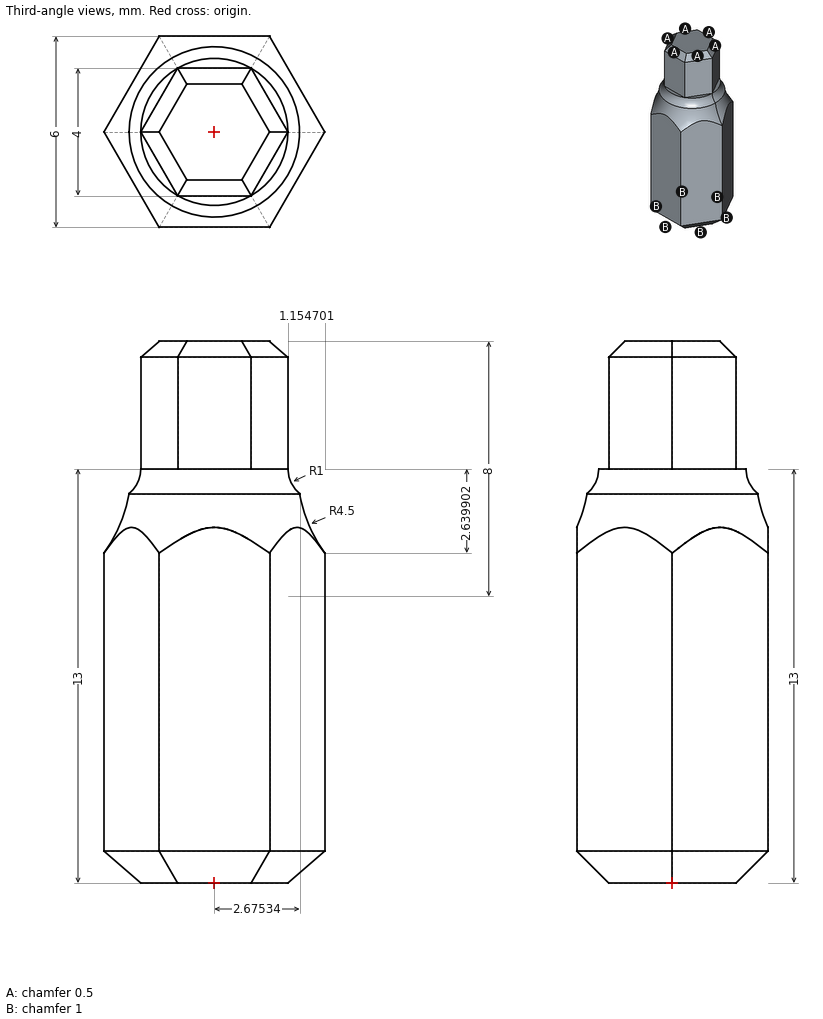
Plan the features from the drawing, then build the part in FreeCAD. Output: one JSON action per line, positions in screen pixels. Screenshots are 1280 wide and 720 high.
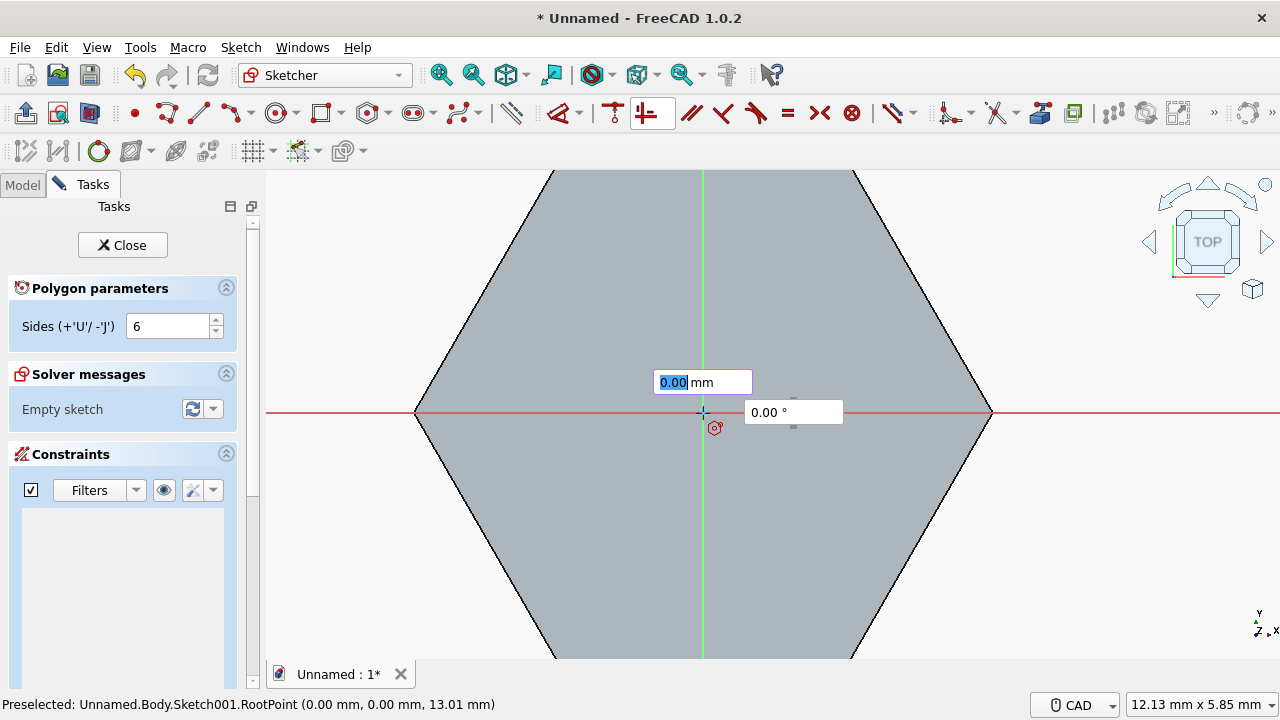
{"action": "left_click", "coordinate": [896, 413]}
{"action": "right_click", "coordinate": [896, 413]}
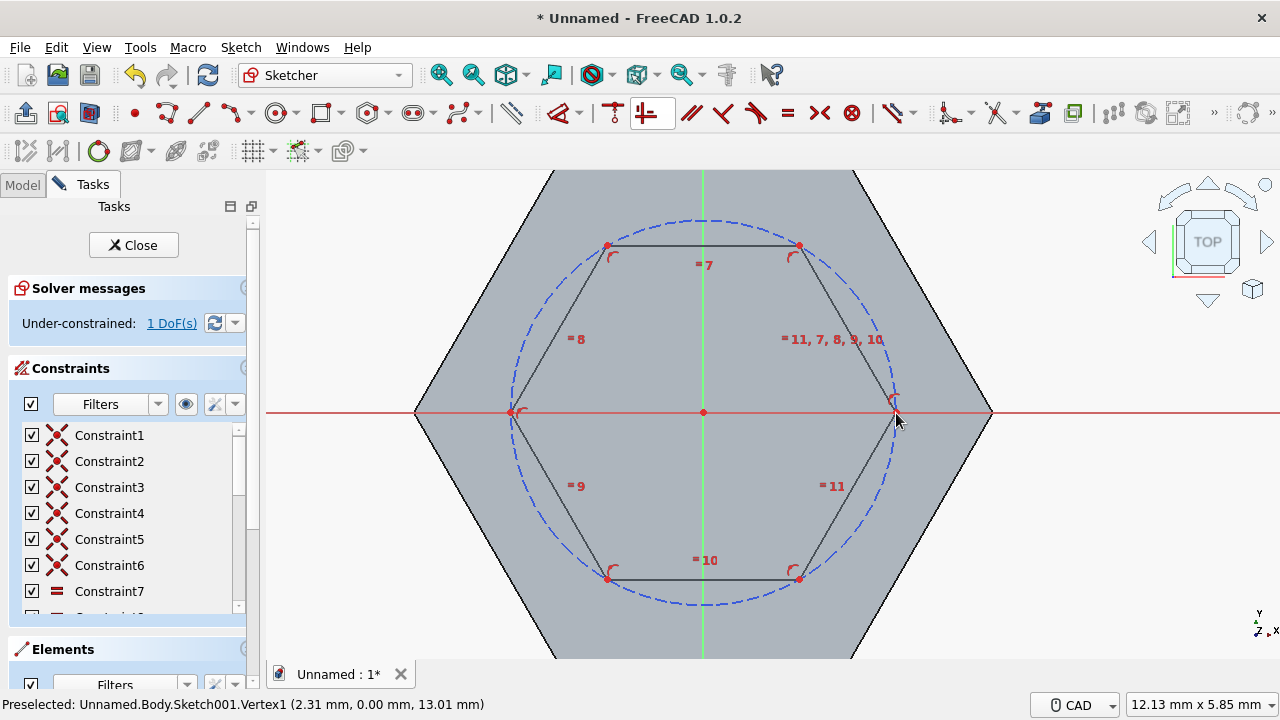
{"action": "left_click", "coordinate": [558, 114]}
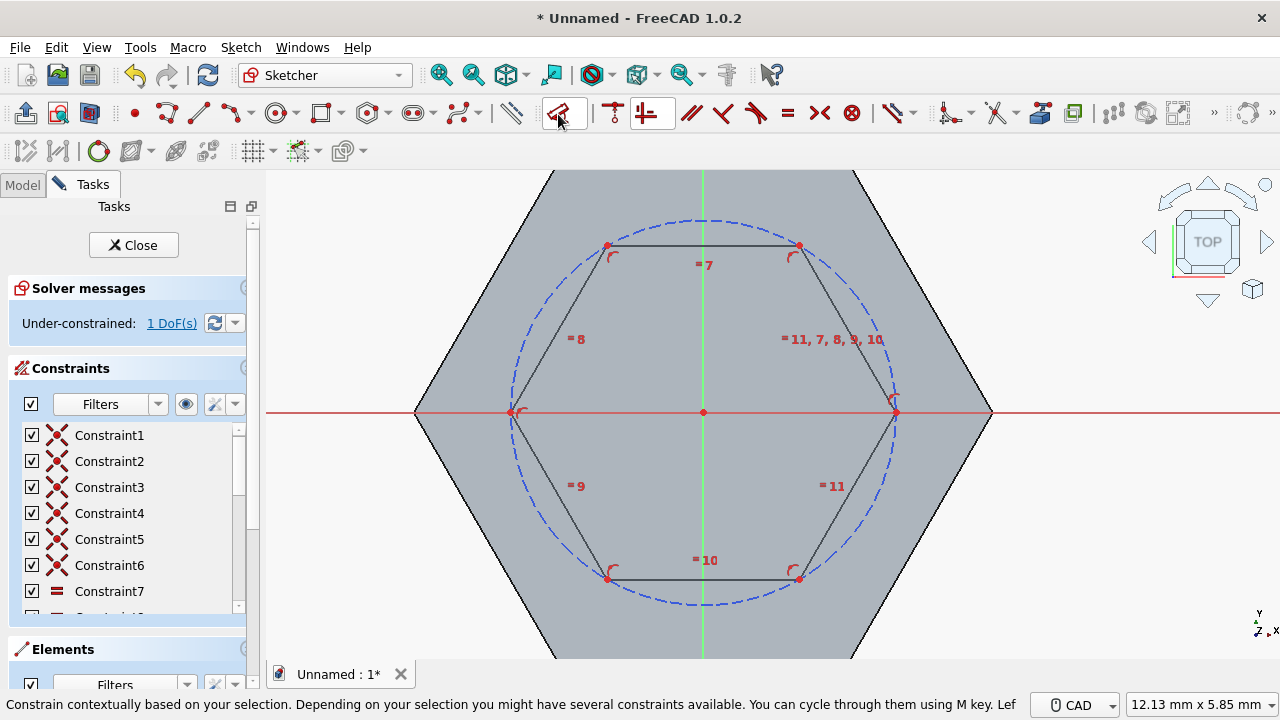
{"action": "left_click", "coordinate": [607, 580]}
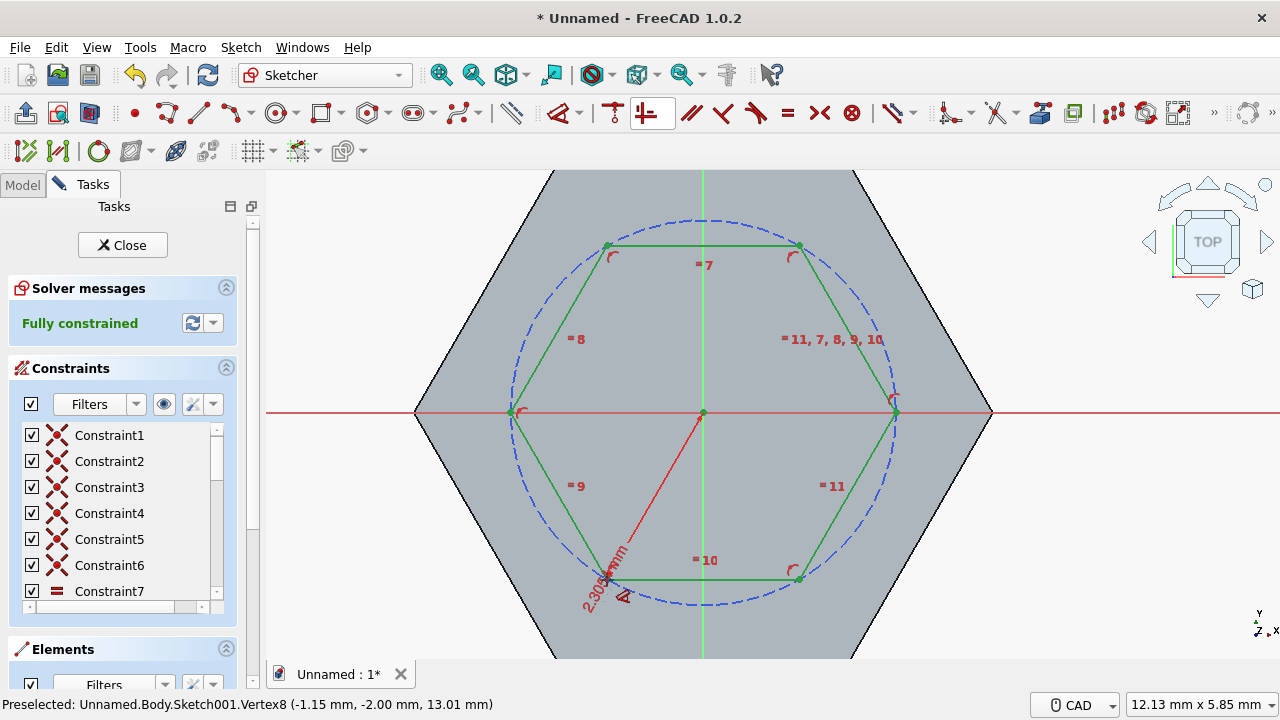
{"action": "left_click", "coordinate": [800, 246]}
{"action": "left_click", "coordinate": [834, 336]}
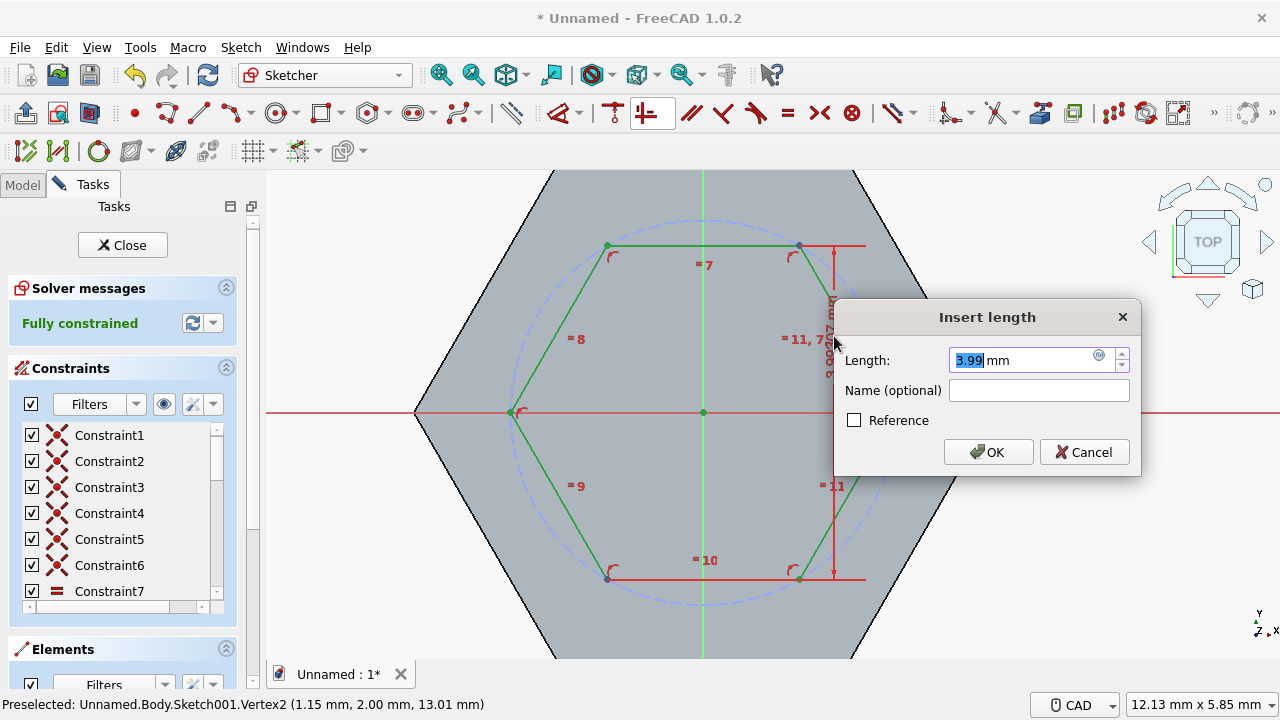
{"action": "type", "text": "4"}
{"action": "key", "text": "Return"}
{"action": "key", "text": "Escape"}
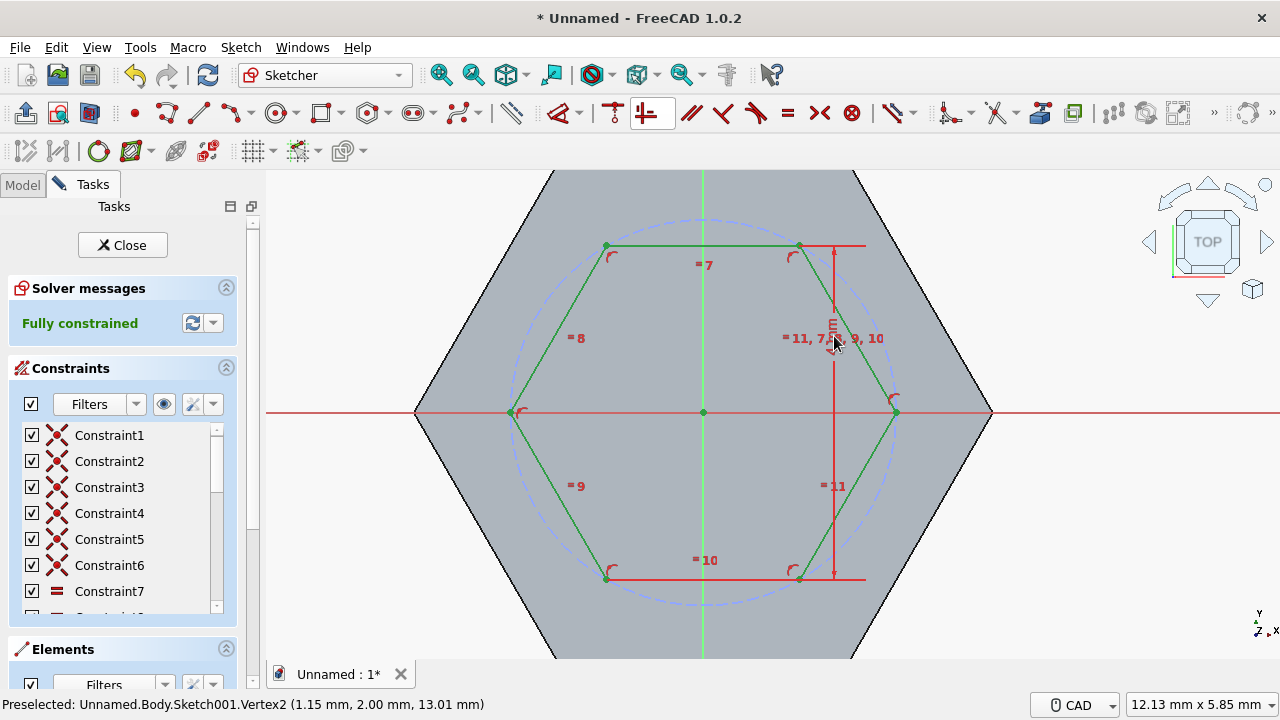
{"action": "left_click", "coordinate": [123, 245]}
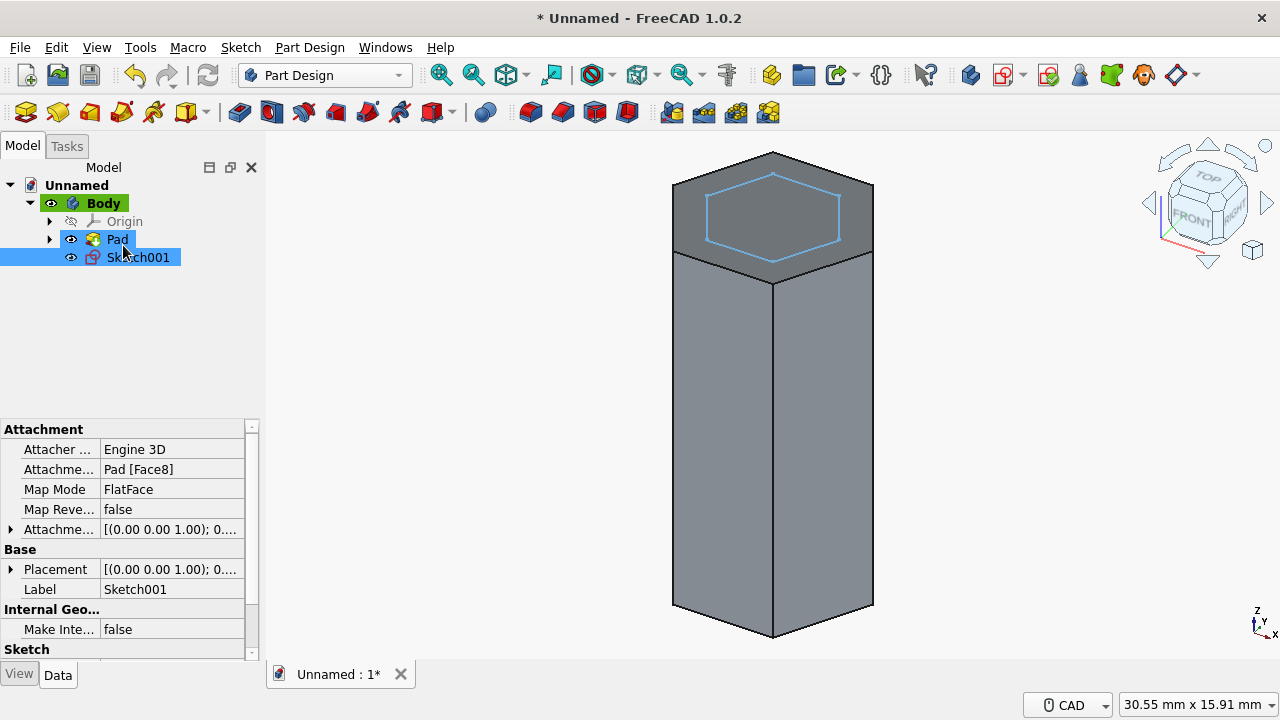
{"action": "left_click", "coordinate": [26, 112]}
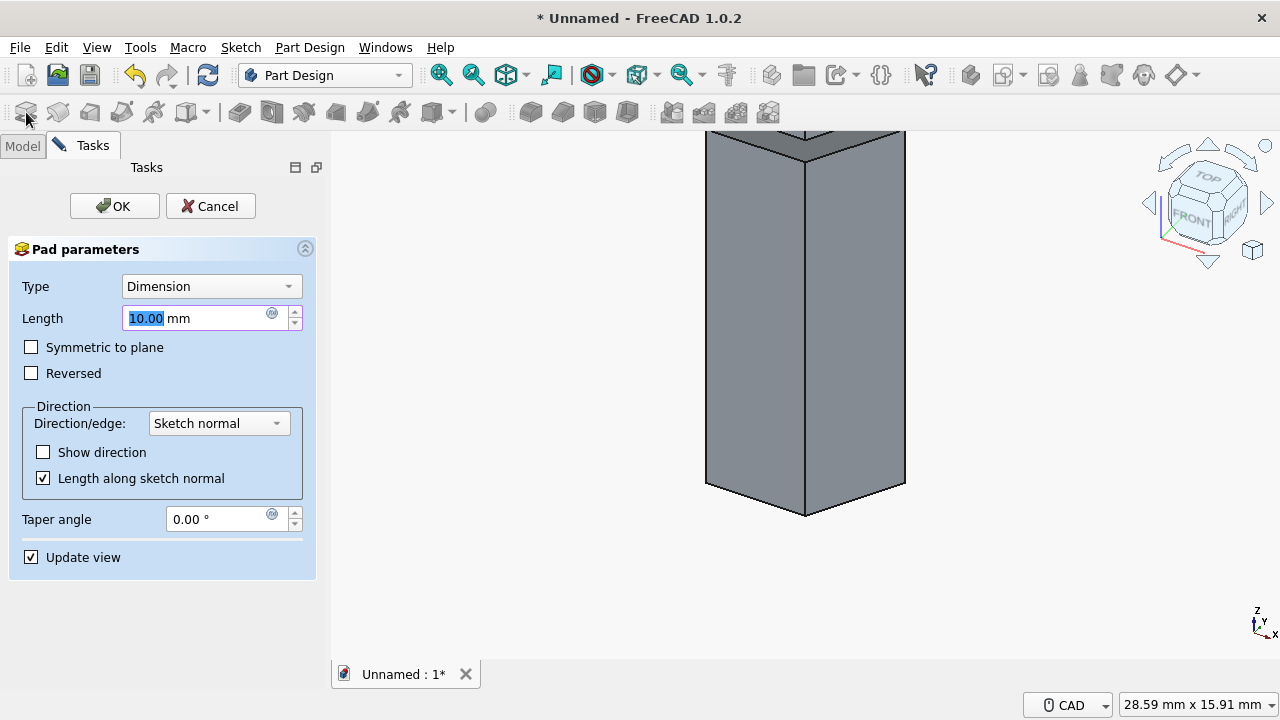
{"action": "type", "text": "8"}
{"action": "key", "text": "Tab"}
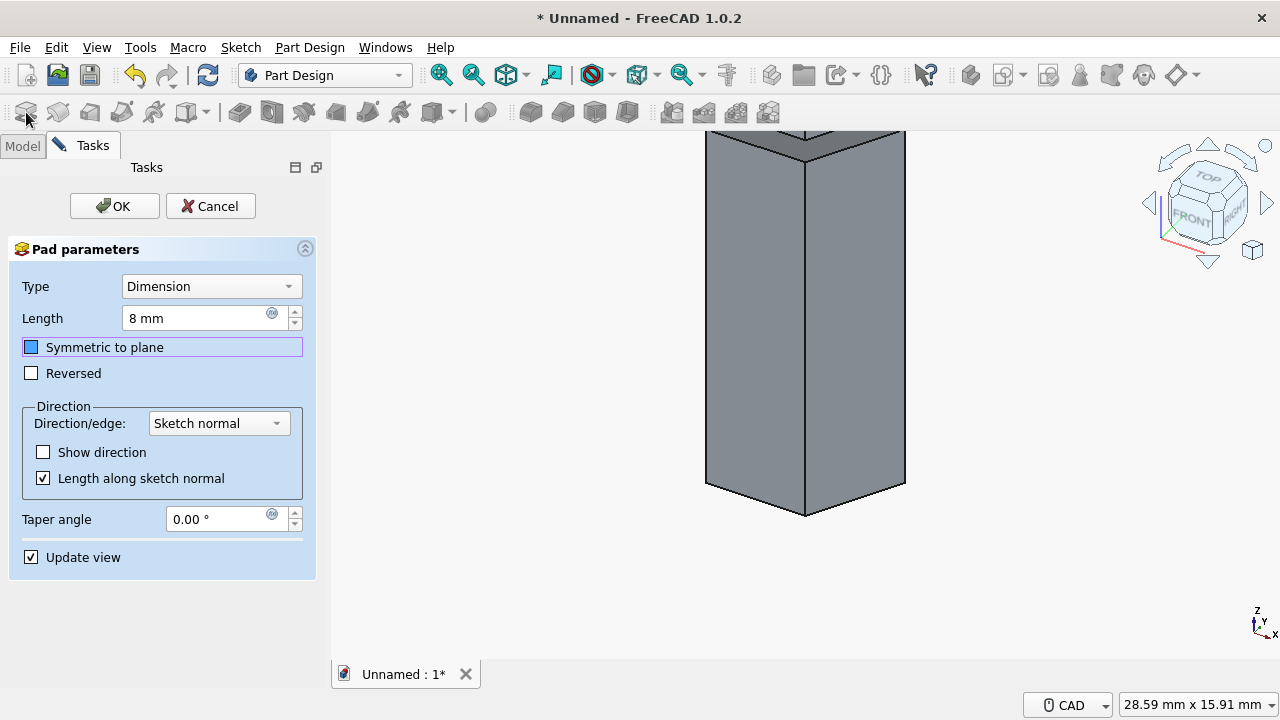
{"action": "left_click", "coordinate": [30, 347]}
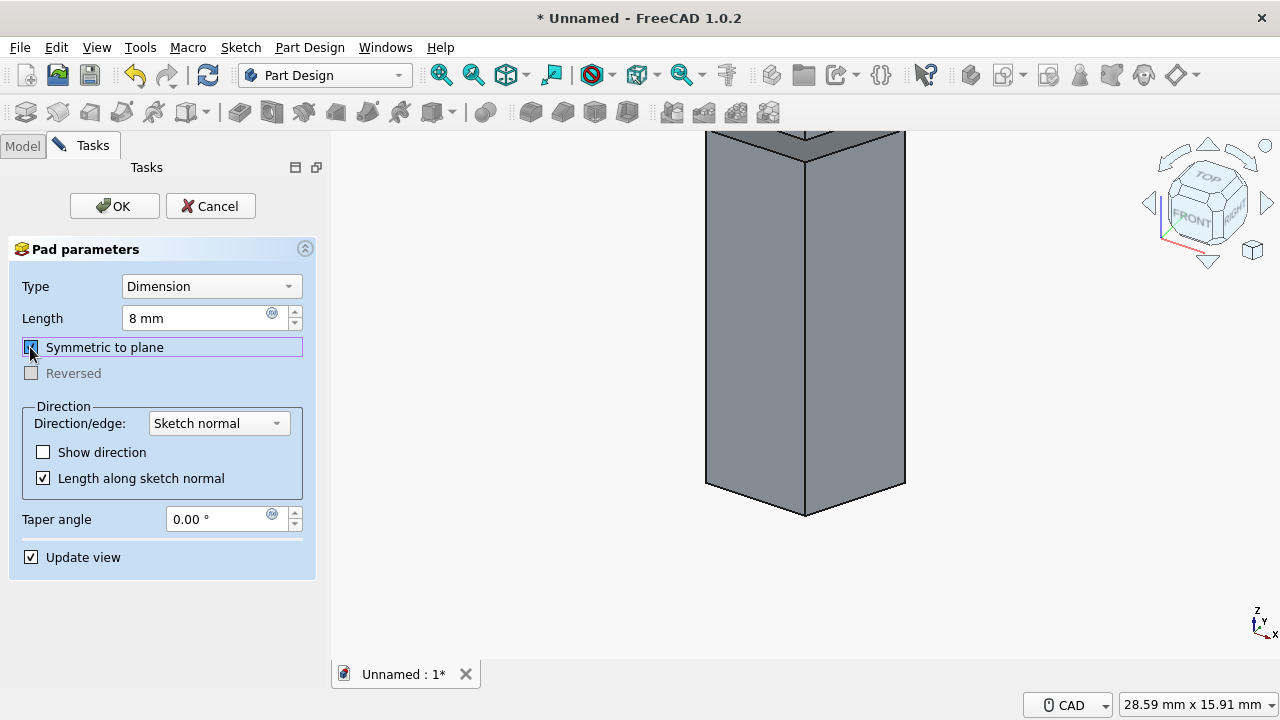
{"action": "left_click", "coordinate": [115, 206]}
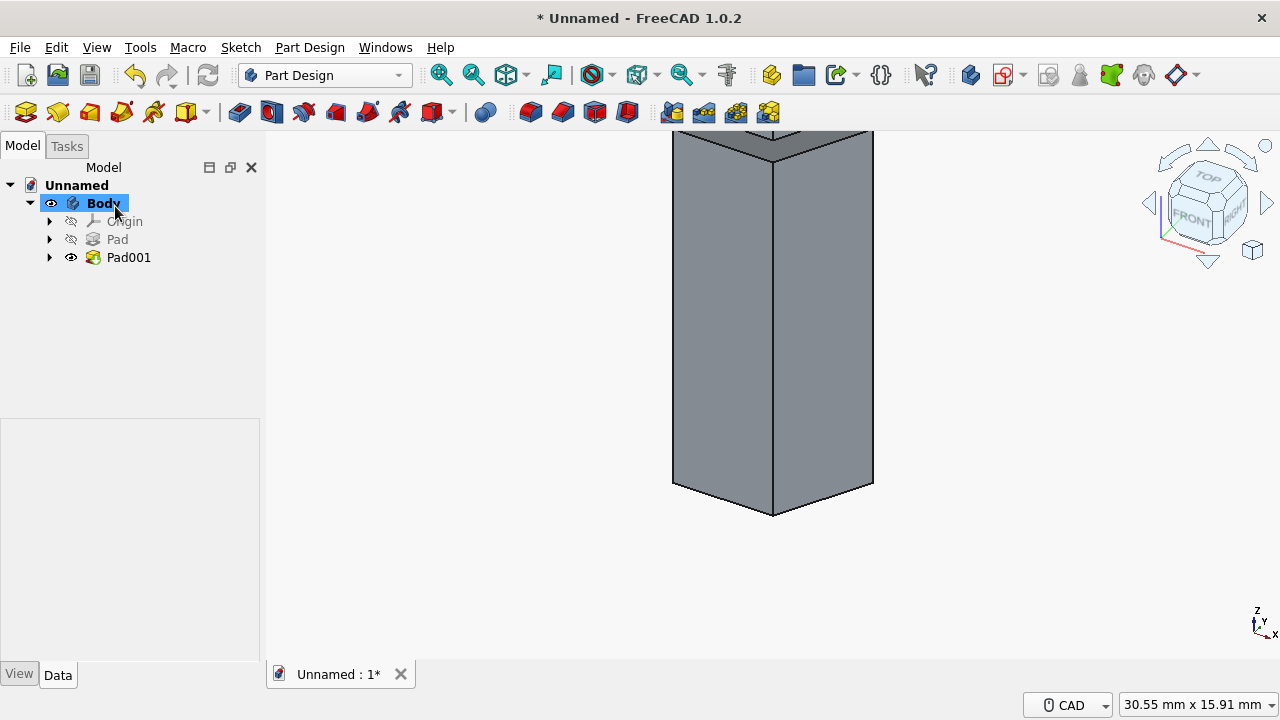
{"action": "left_click", "coordinate": [442, 76]}